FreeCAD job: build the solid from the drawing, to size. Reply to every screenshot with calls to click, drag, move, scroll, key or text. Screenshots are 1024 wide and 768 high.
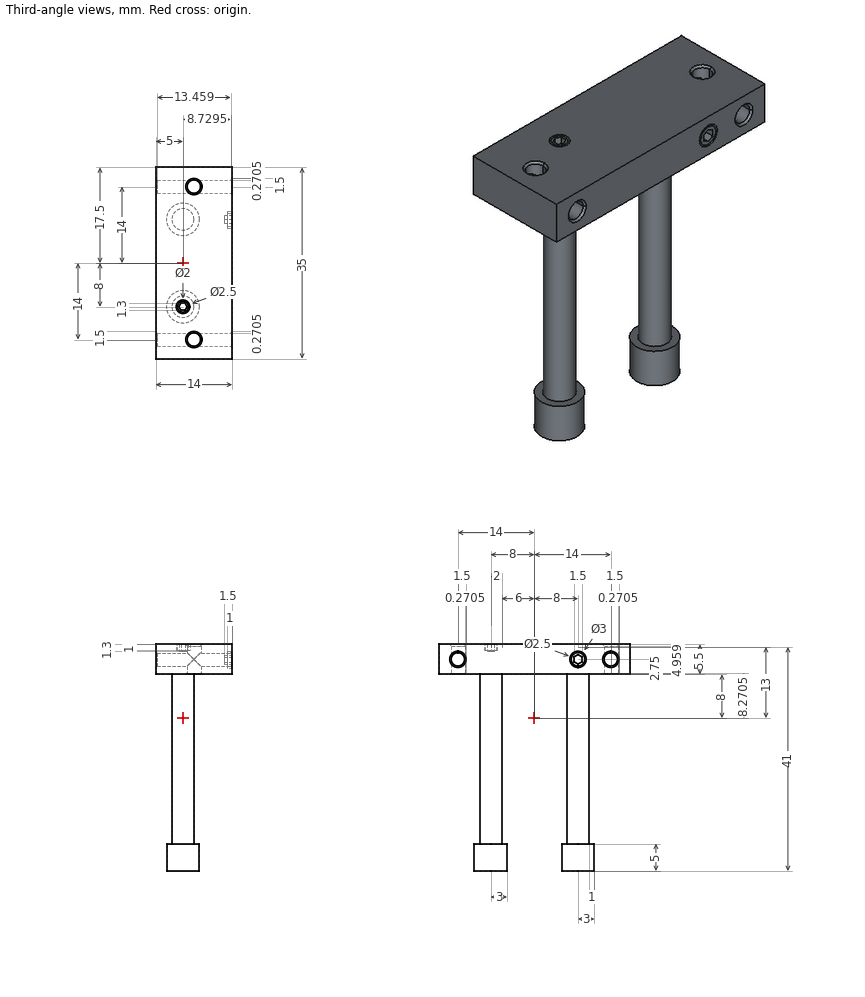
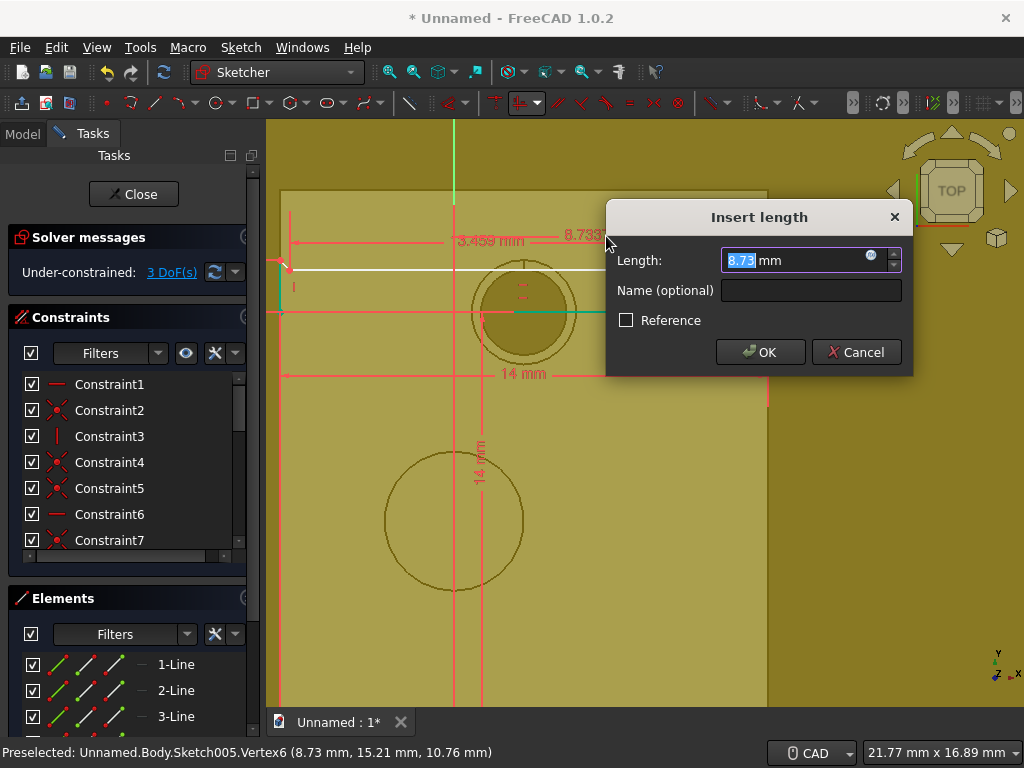
text(8.7295)
key(Return)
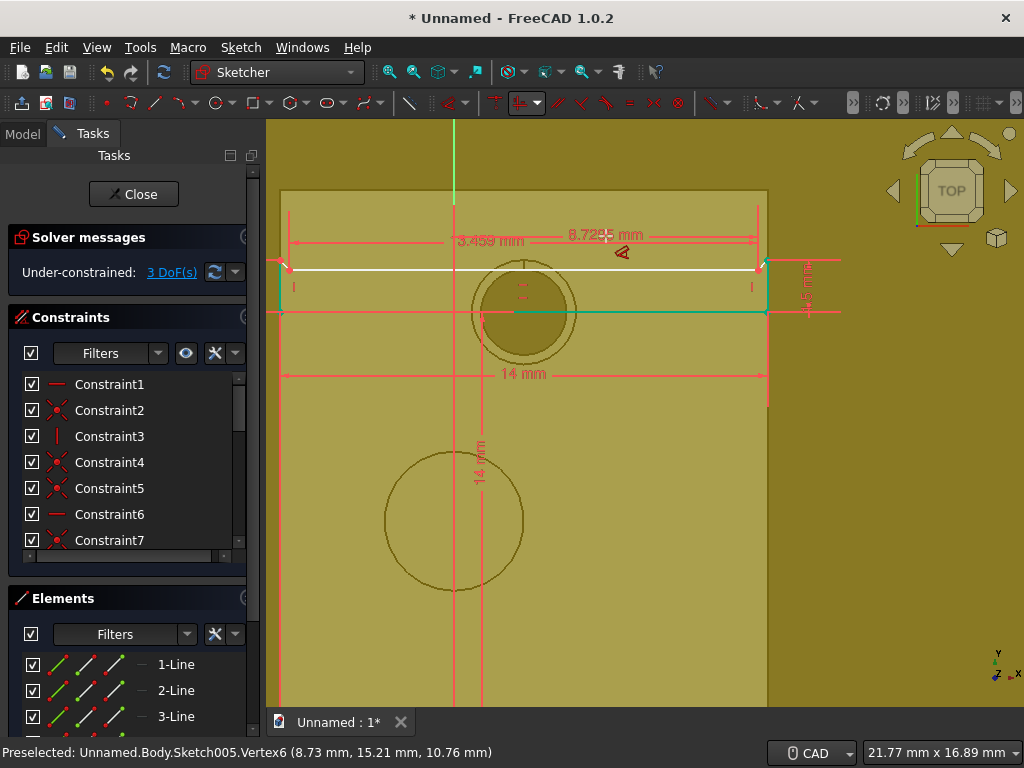
scroll(762, 266, up, 8)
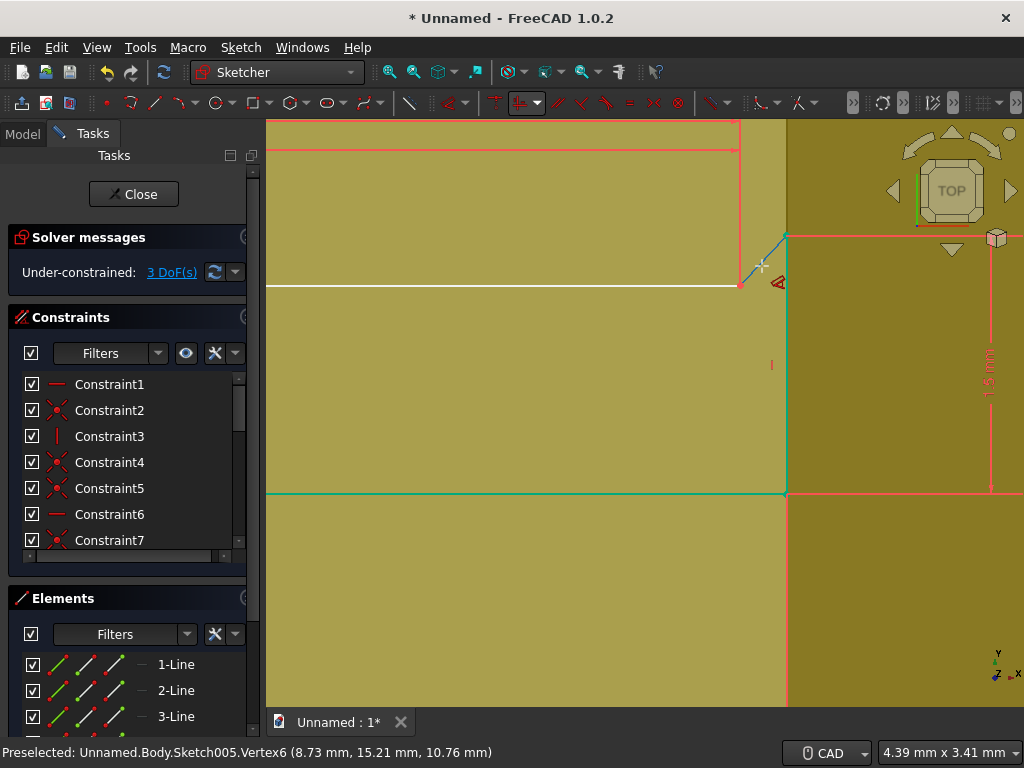
click(759, 266)
click(821, 261)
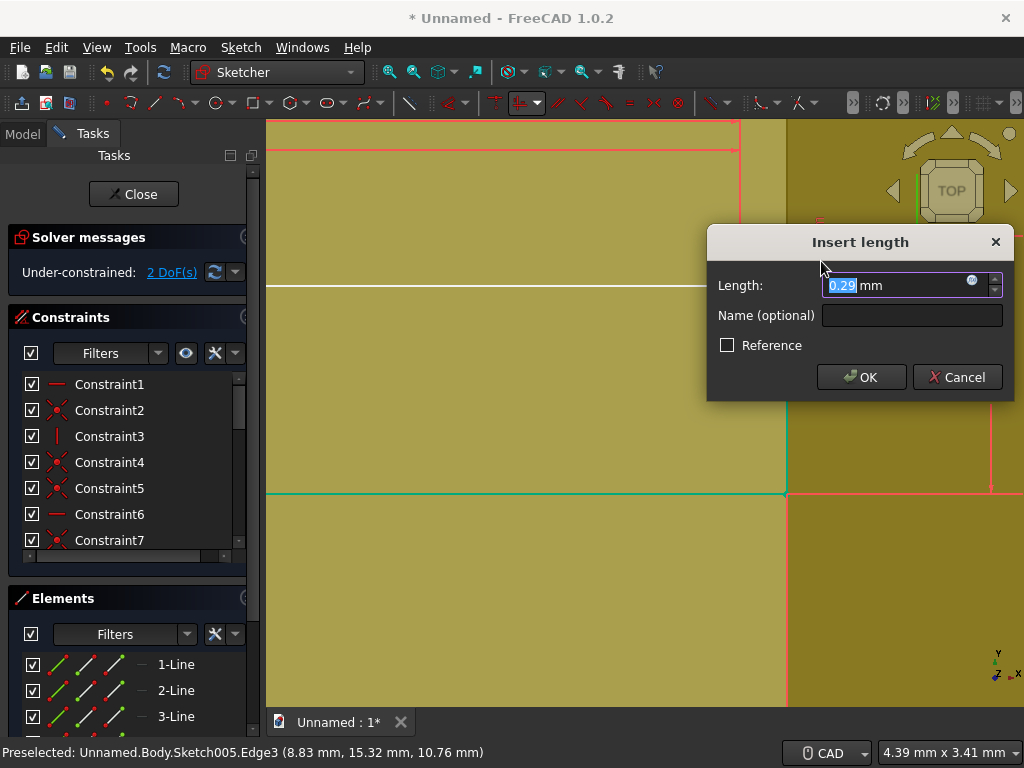
text(0.2705)
key(Return)
key(Escape)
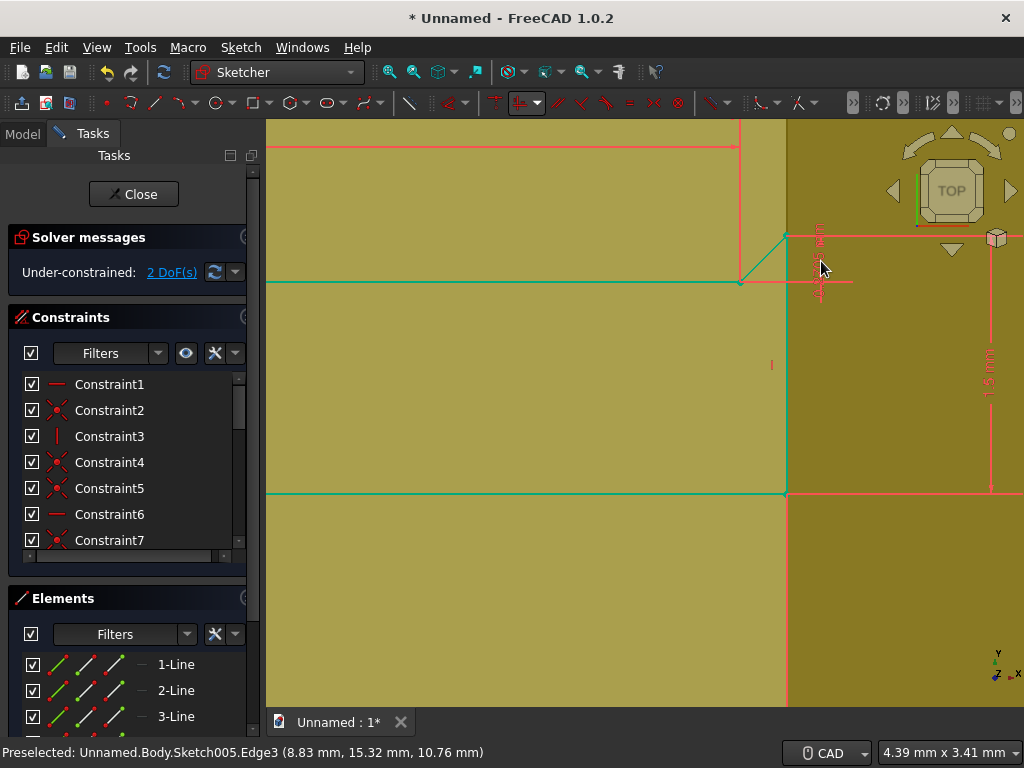
click(134, 194)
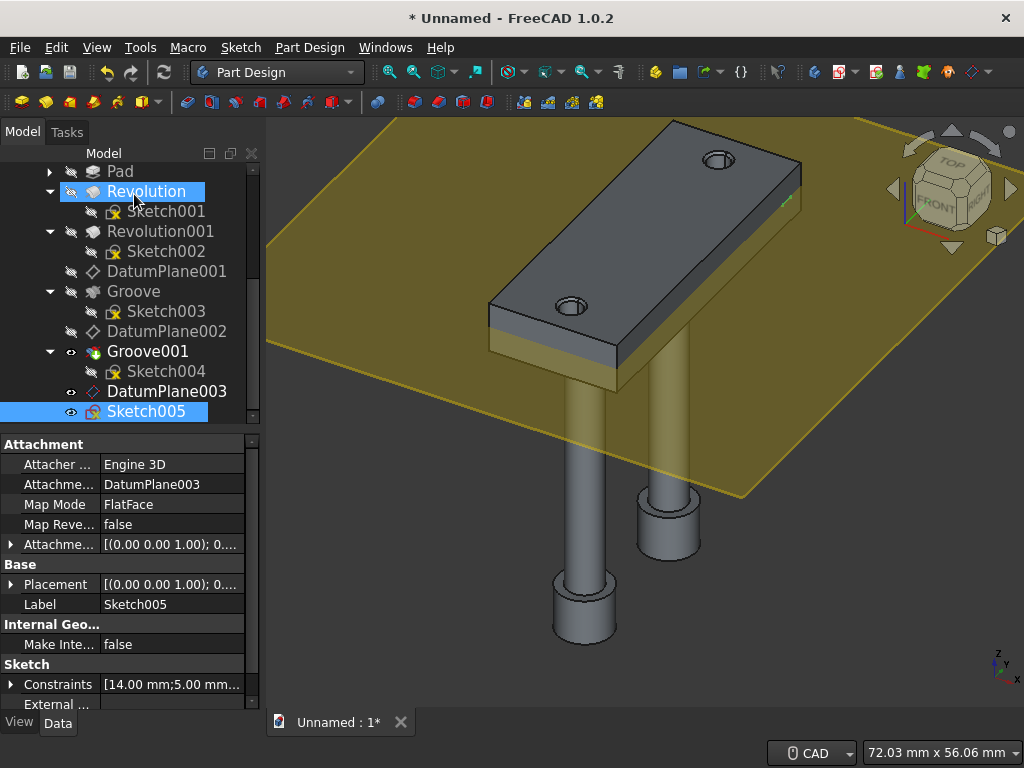
click(236, 102)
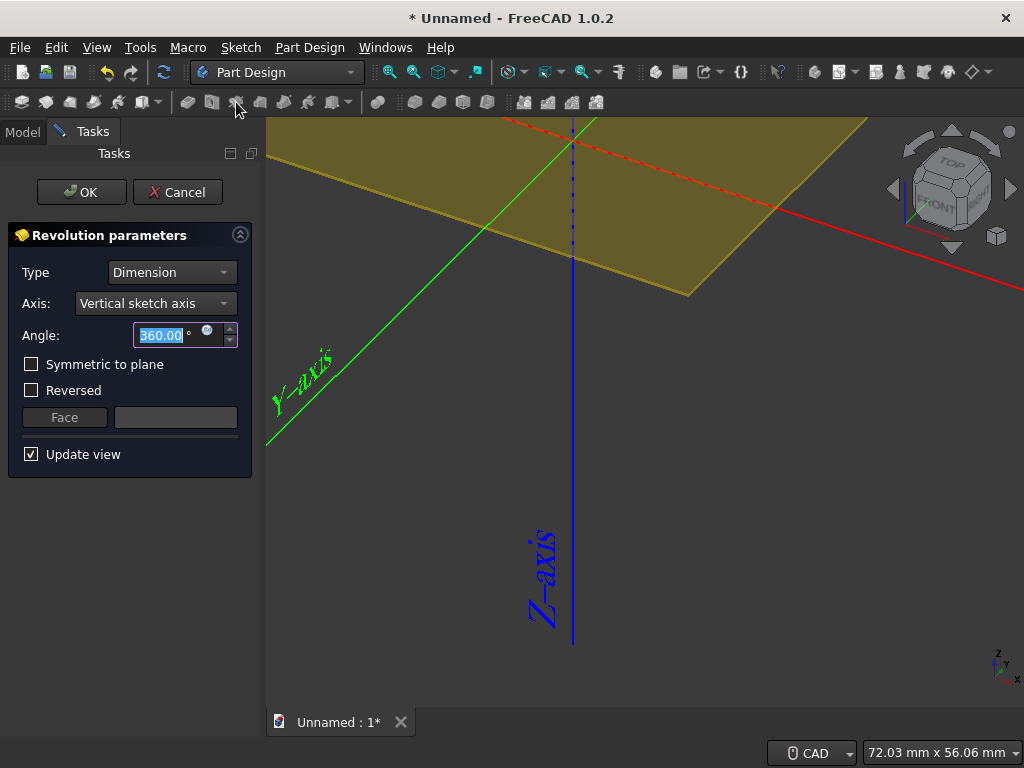
click(156, 304)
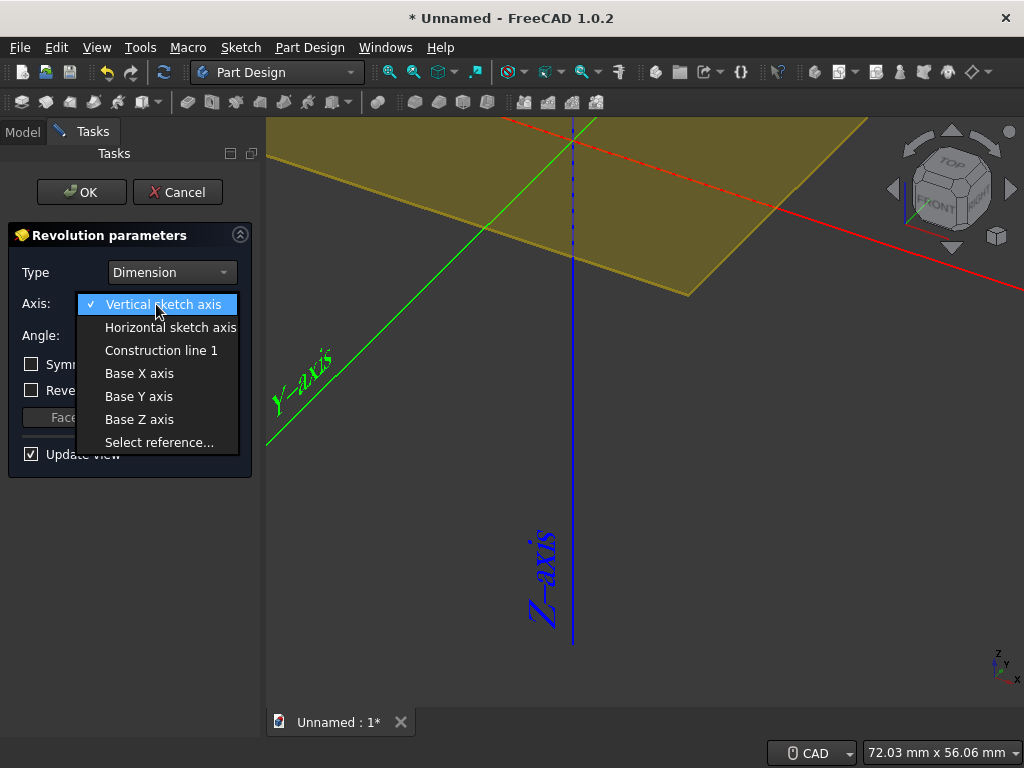
click(156, 350)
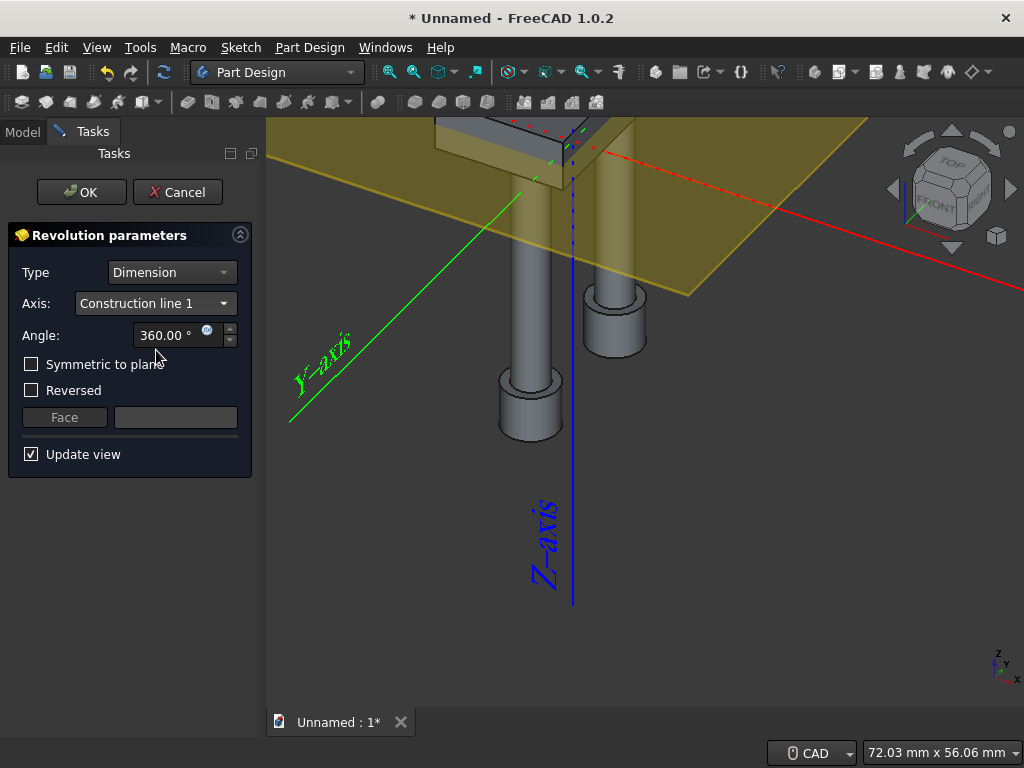
click(82, 192)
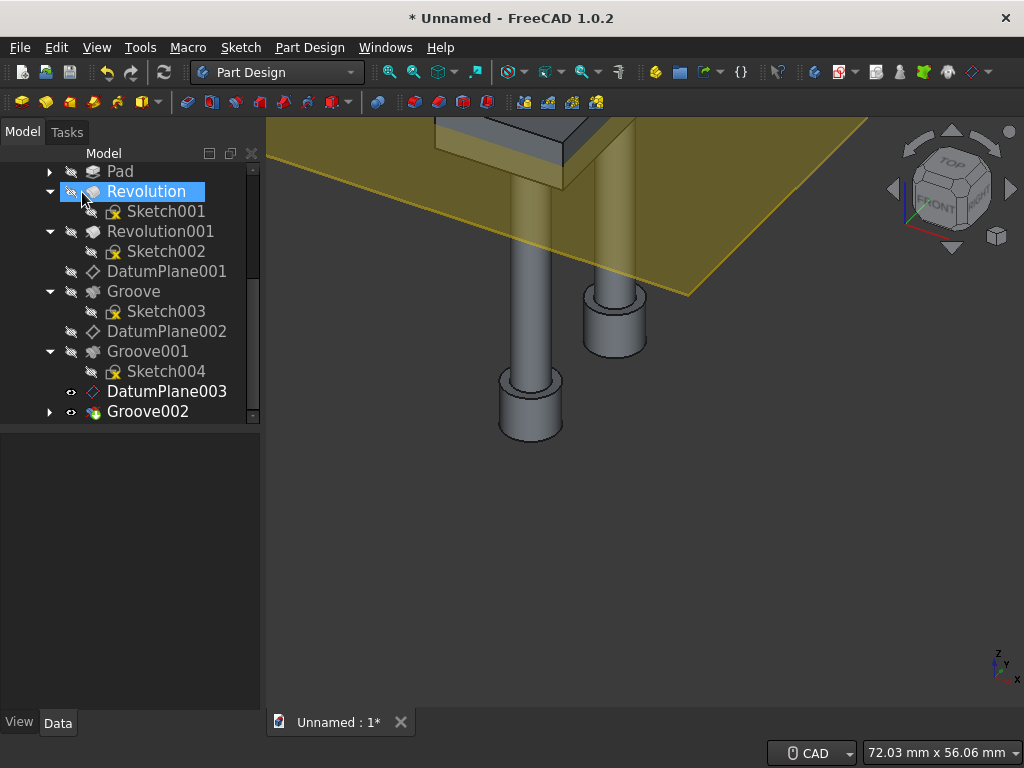
click(116, 392)
key(space)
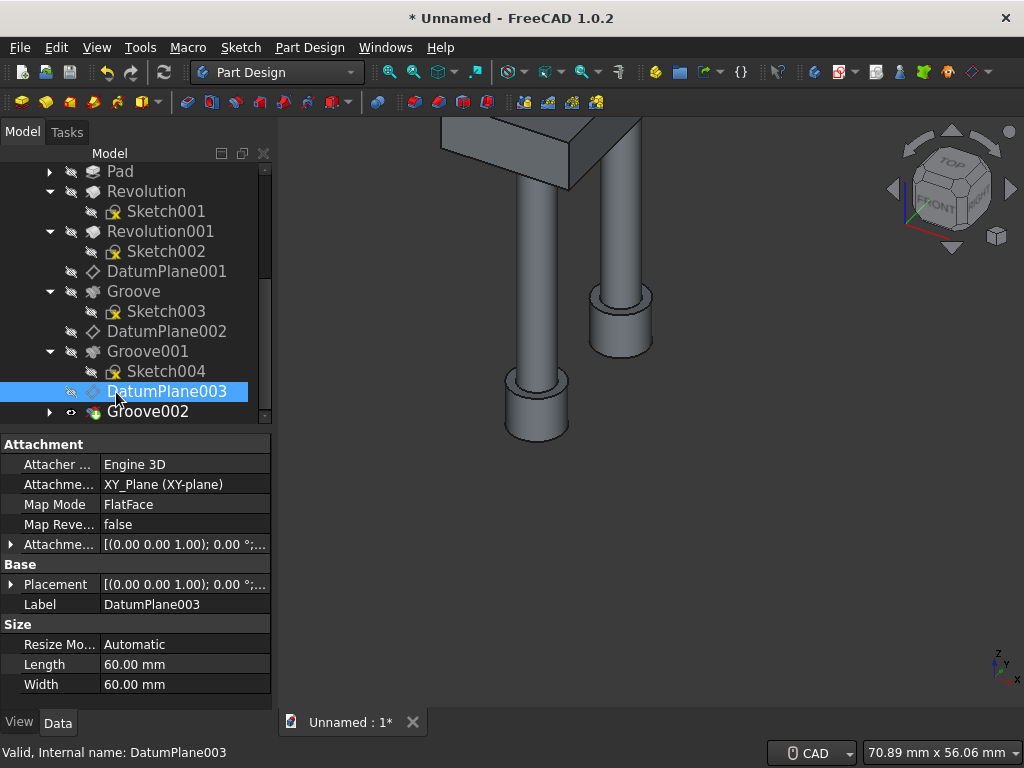
click(390, 72)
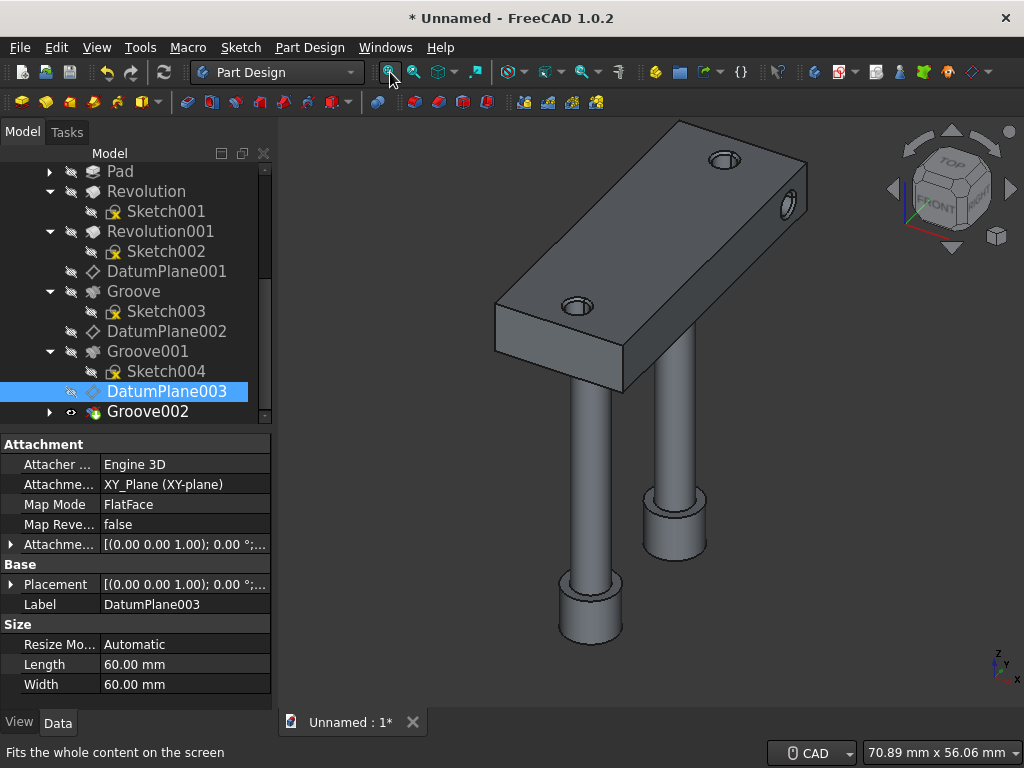
scroll(140, 287, down, 3)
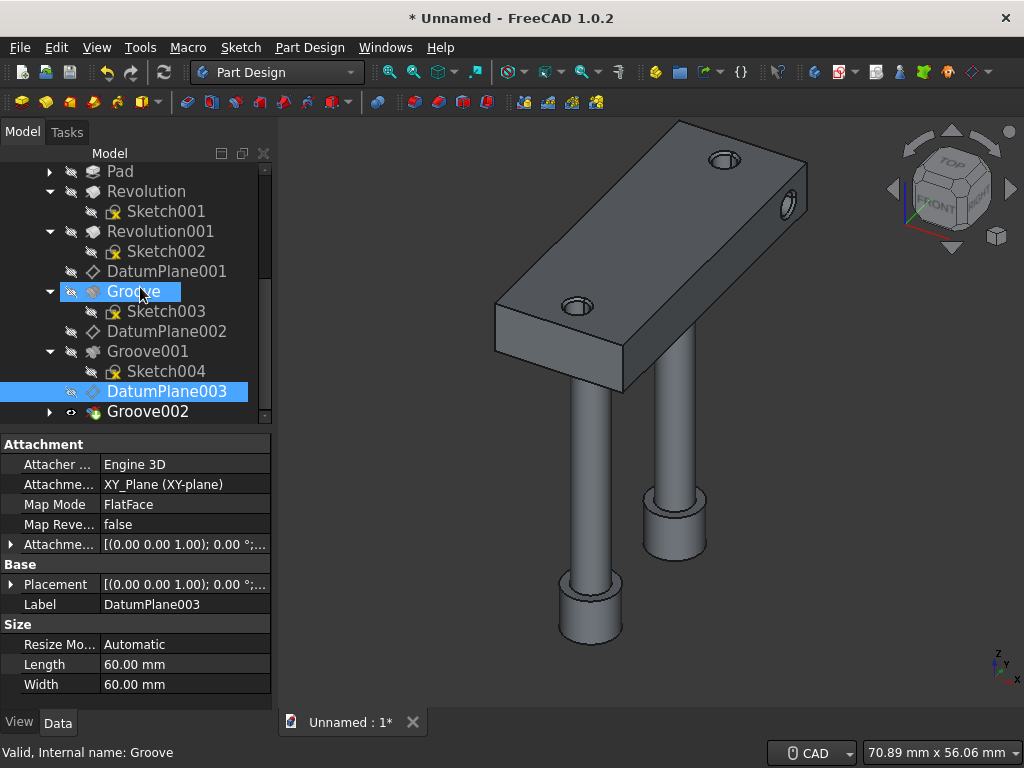
scroll(140, 287, up, 15)